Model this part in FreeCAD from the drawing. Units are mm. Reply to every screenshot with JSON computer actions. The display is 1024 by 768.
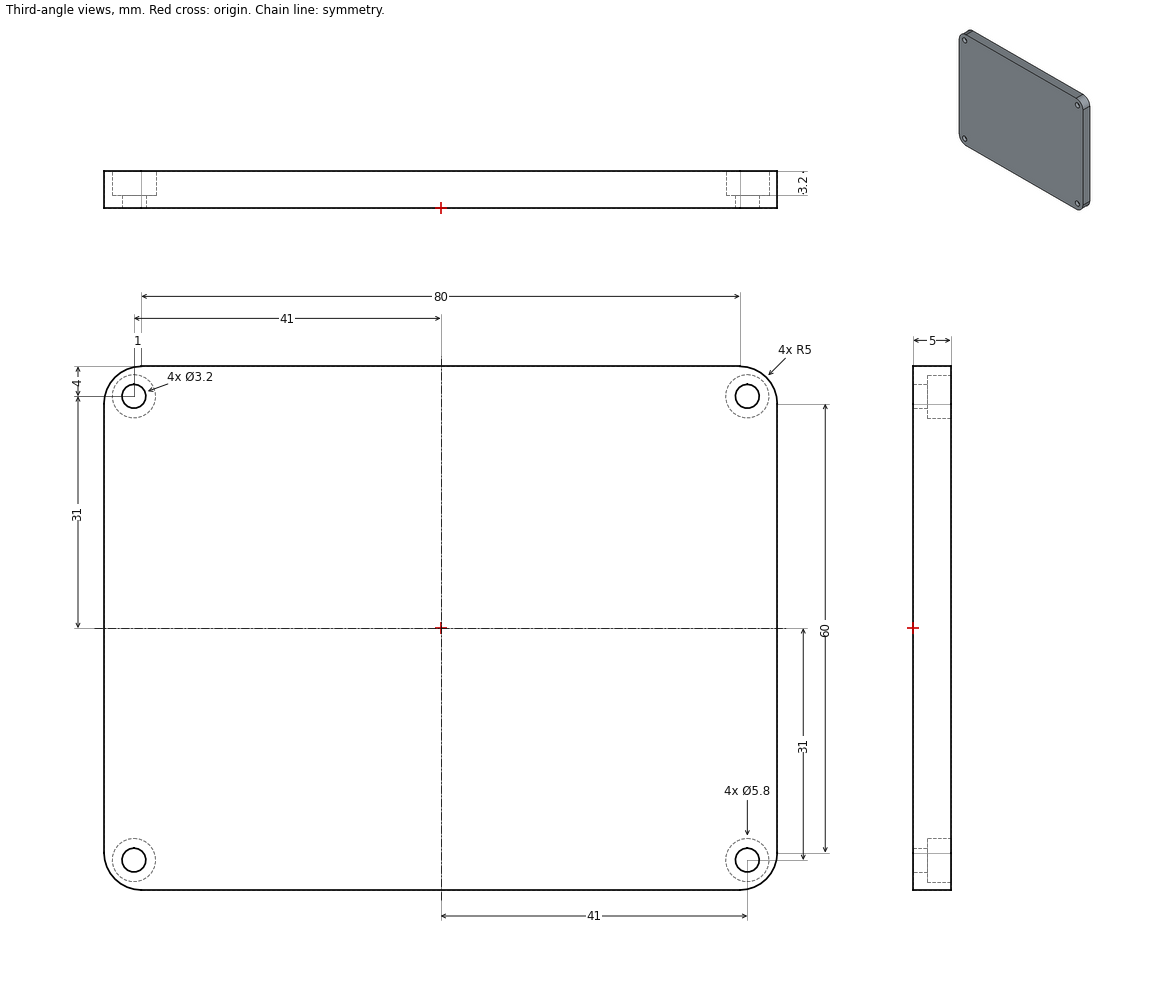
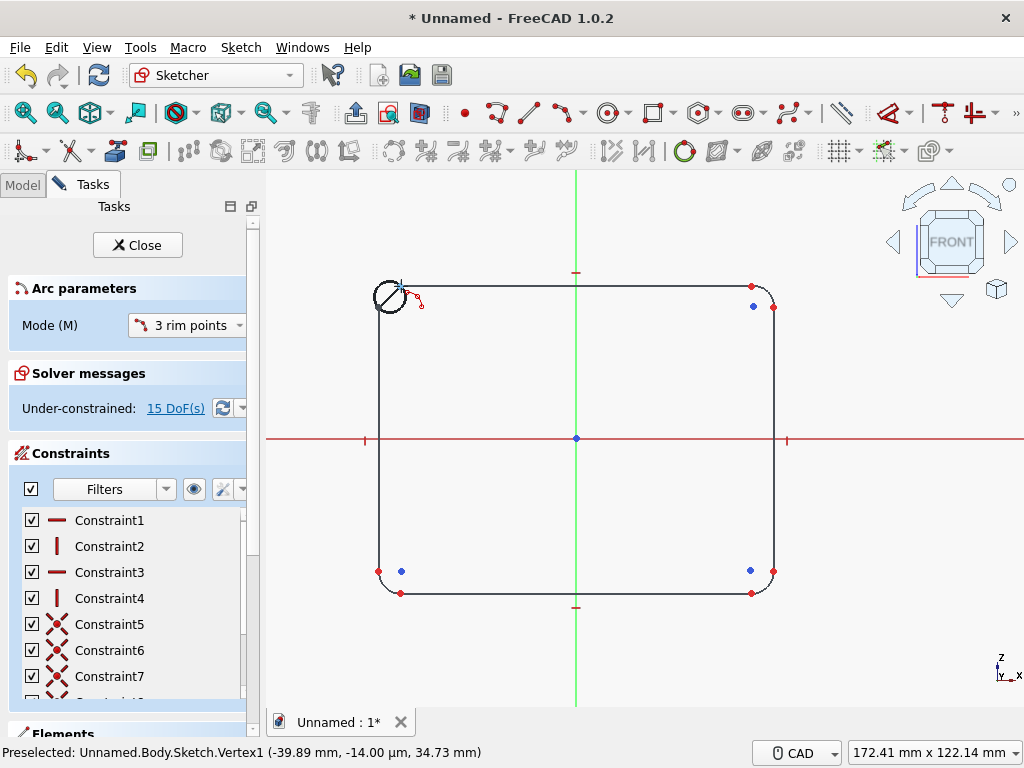
{"action": "scroll", "coordinate": [385, 291], "scroll_direction": "up", "scroll_amount": 5}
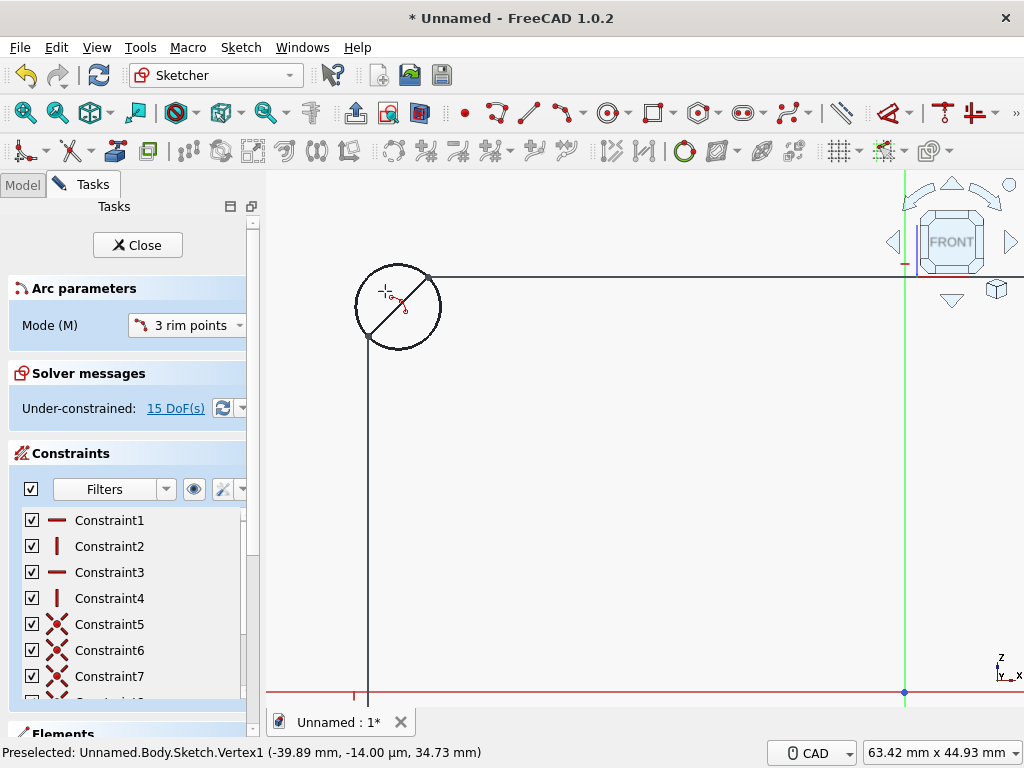
{"action": "left_click", "coordinate": [384, 291]}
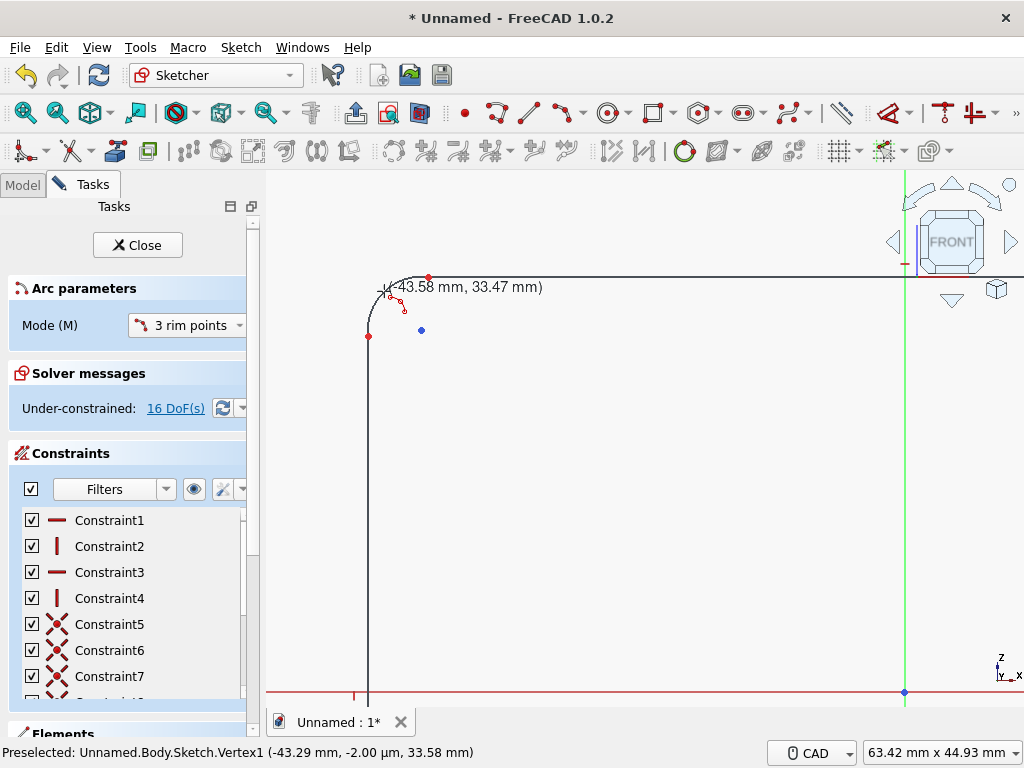
{"action": "key", "text": "g c"}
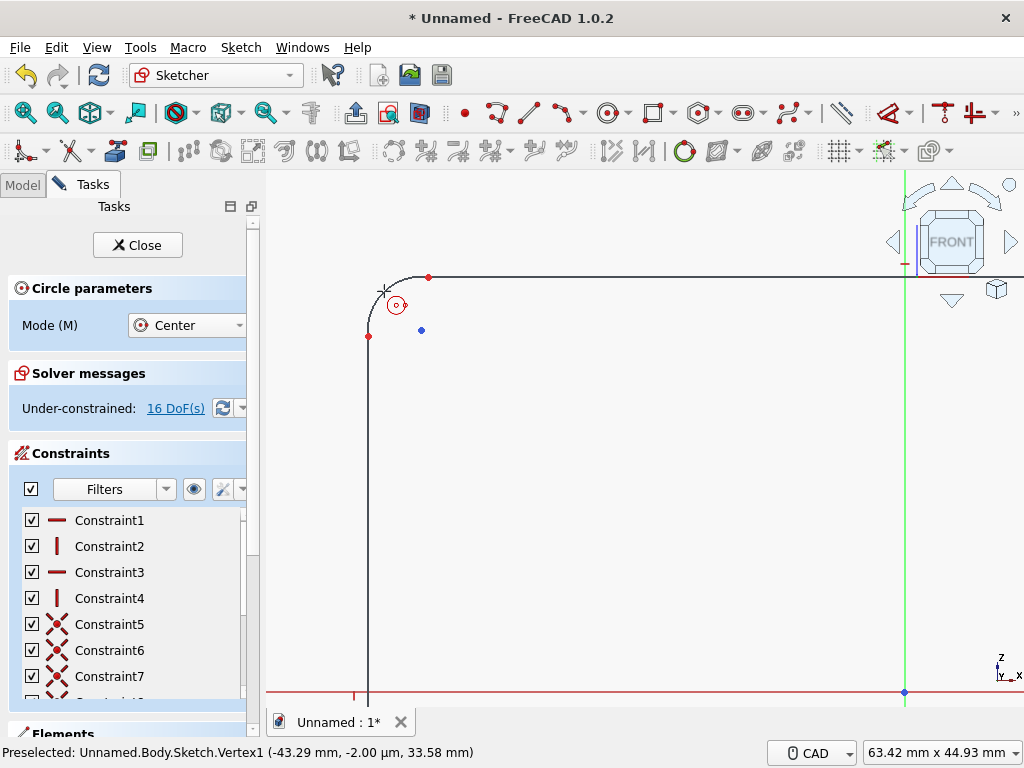
{"action": "left_click", "coordinate": [415, 322]}
{"action": "mouse_move", "coordinate": [428, 308]}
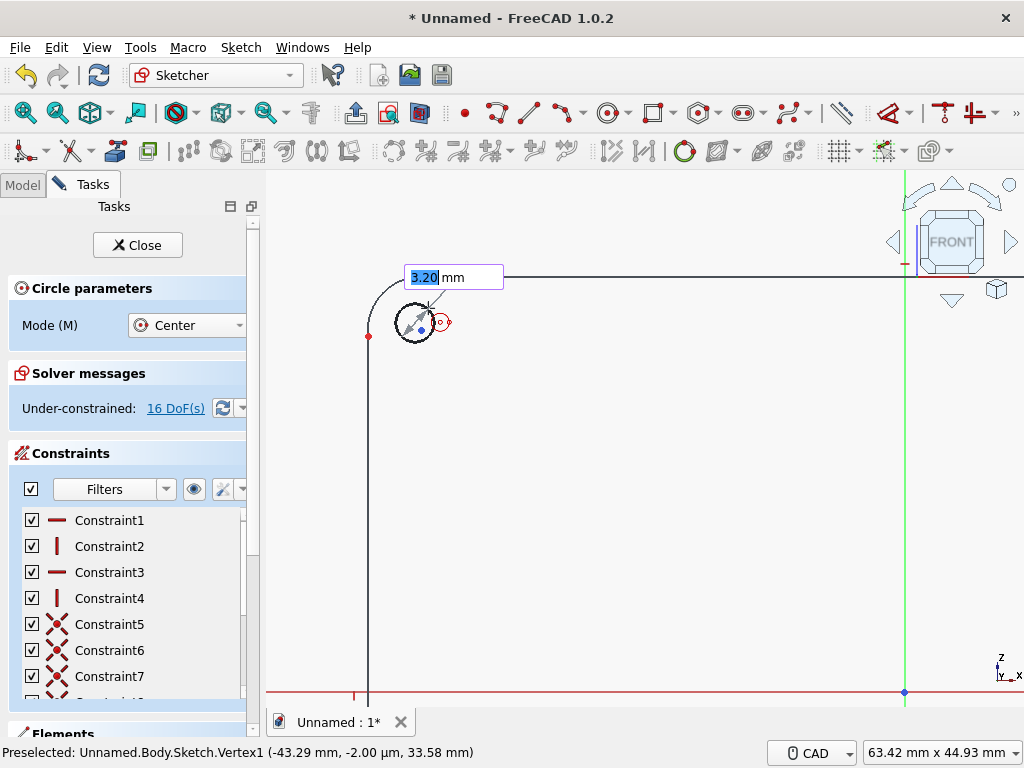
{"action": "type", "text": "3.2"}
{"action": "key", "text": "Return"}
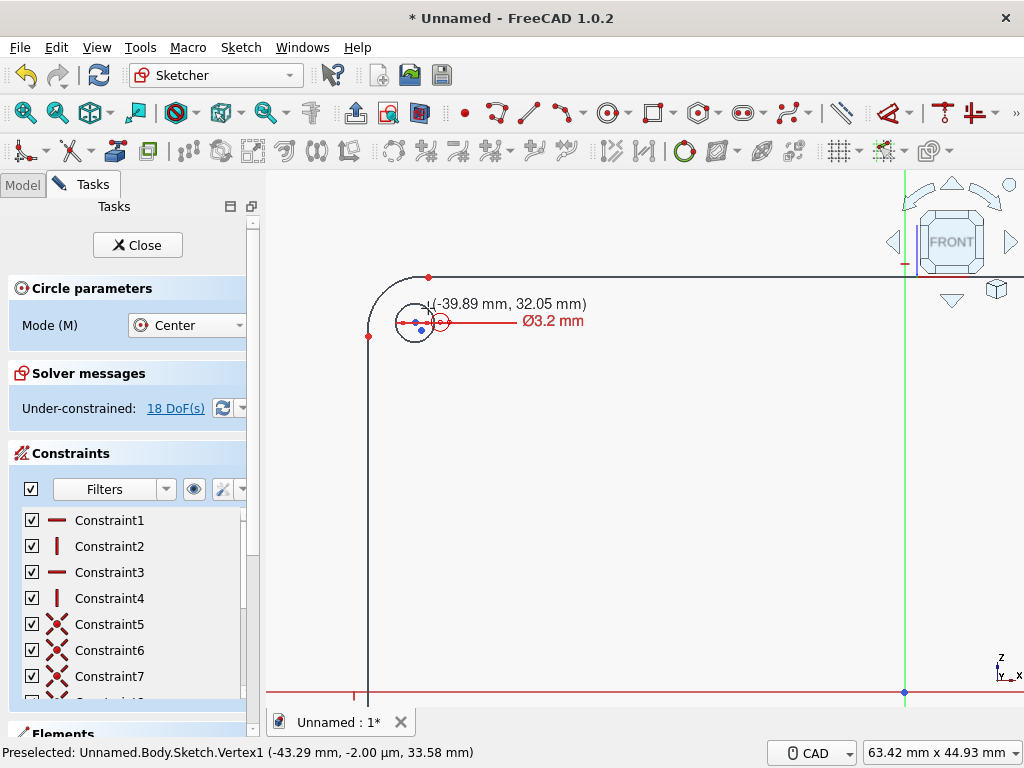
{"action": "scroll", "coordinate": [385, 291], "scroll_direction": "down", "scroll_amount": 5}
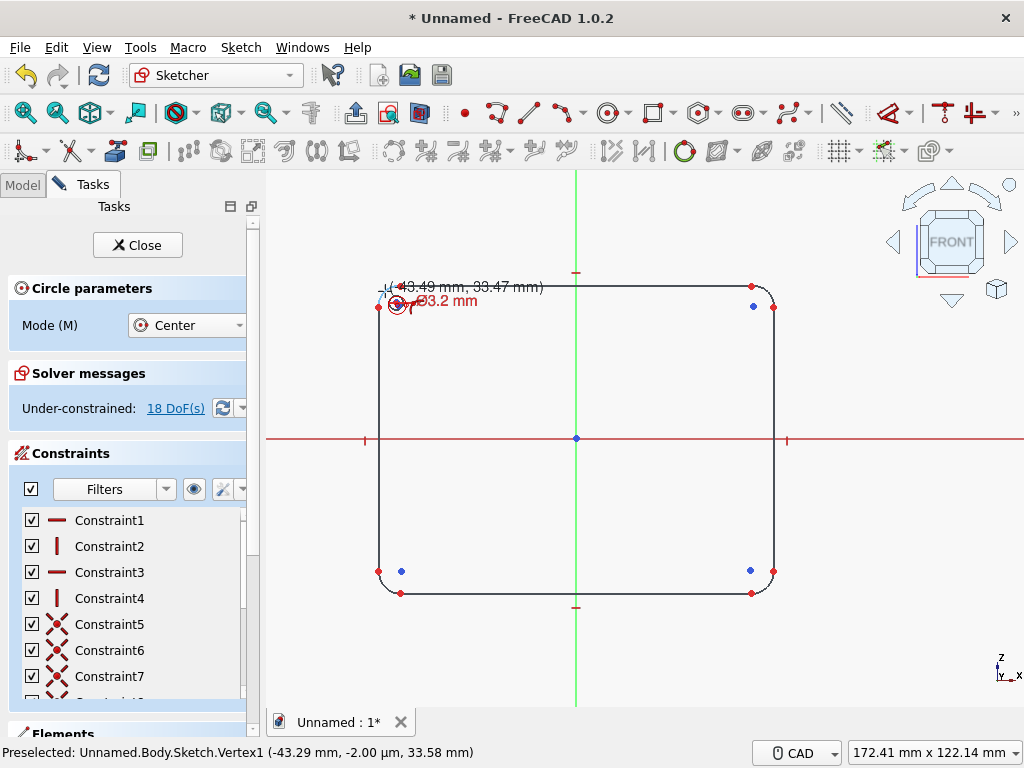
{"action": "scroll", "coordinate": [757, 302], "scroll_direction": "up", "scroll_amount": 6}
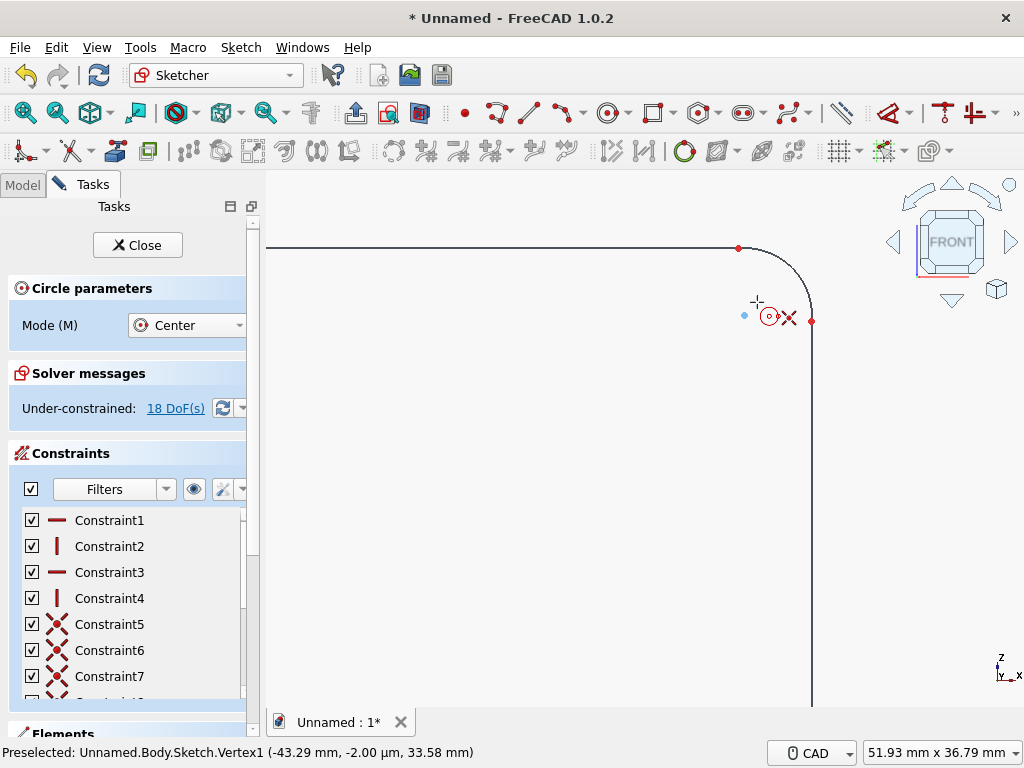
{"action": "left_click", "coordinate": [754, 303]}
{"action": "mouse_move", "coordinate": [771, 286]}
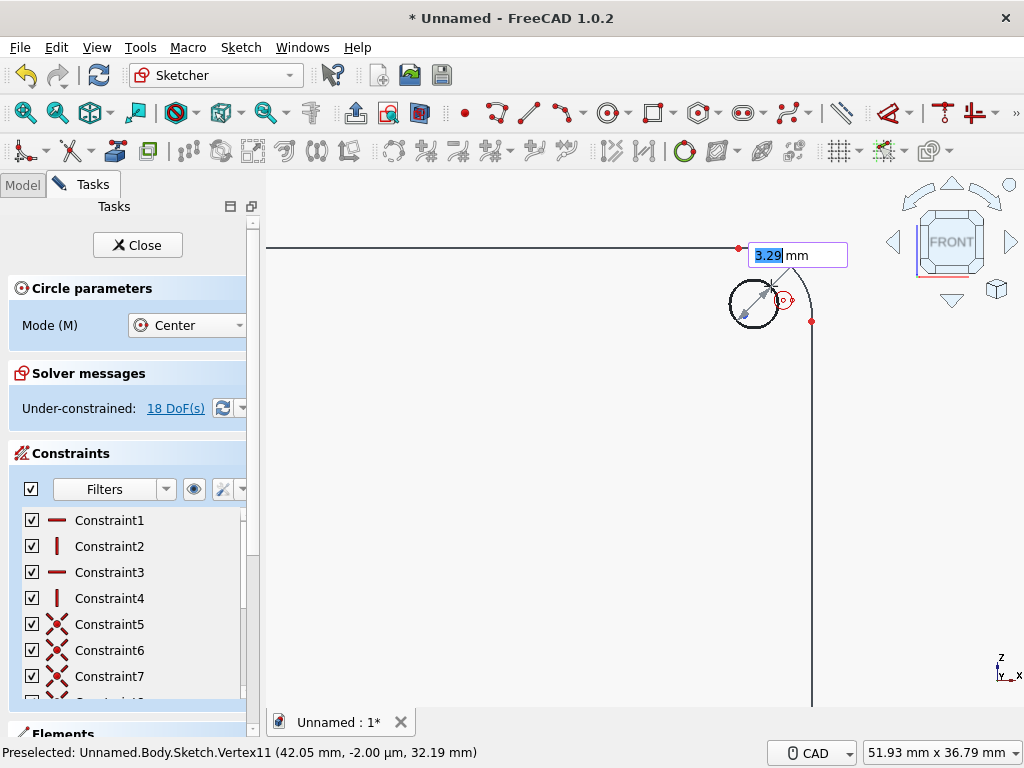
{"action": "type", "text": "3.2"}
{"action": "key", "text": "Return"}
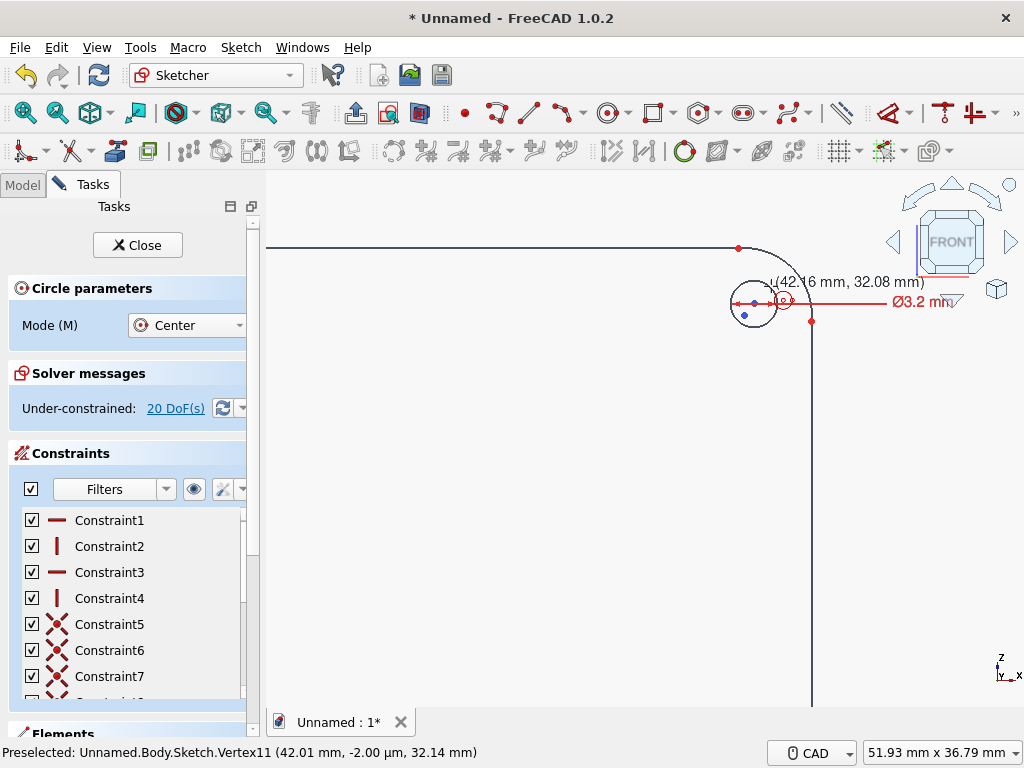
{"action": "scroll", "coordinate": [758, 302], "scroll_direction": "down", "scroll_amount": 6}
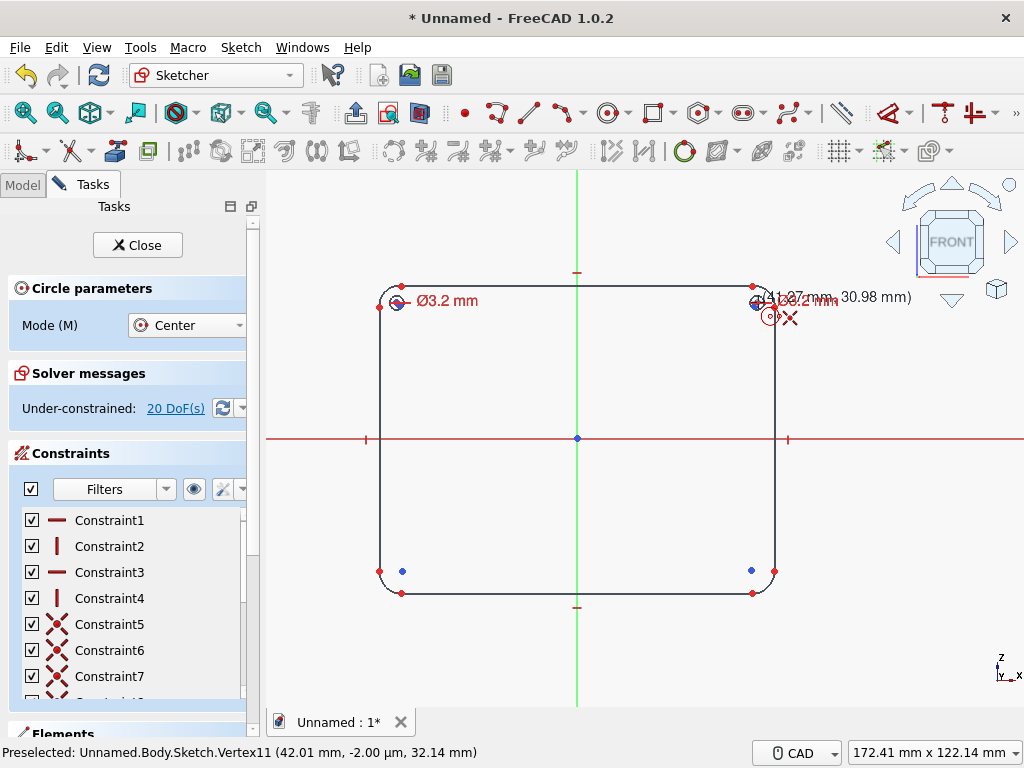
{"action": "scroll", "coordinate": [397, 575], "scroll_direction": "up", "scroll_amount": 6}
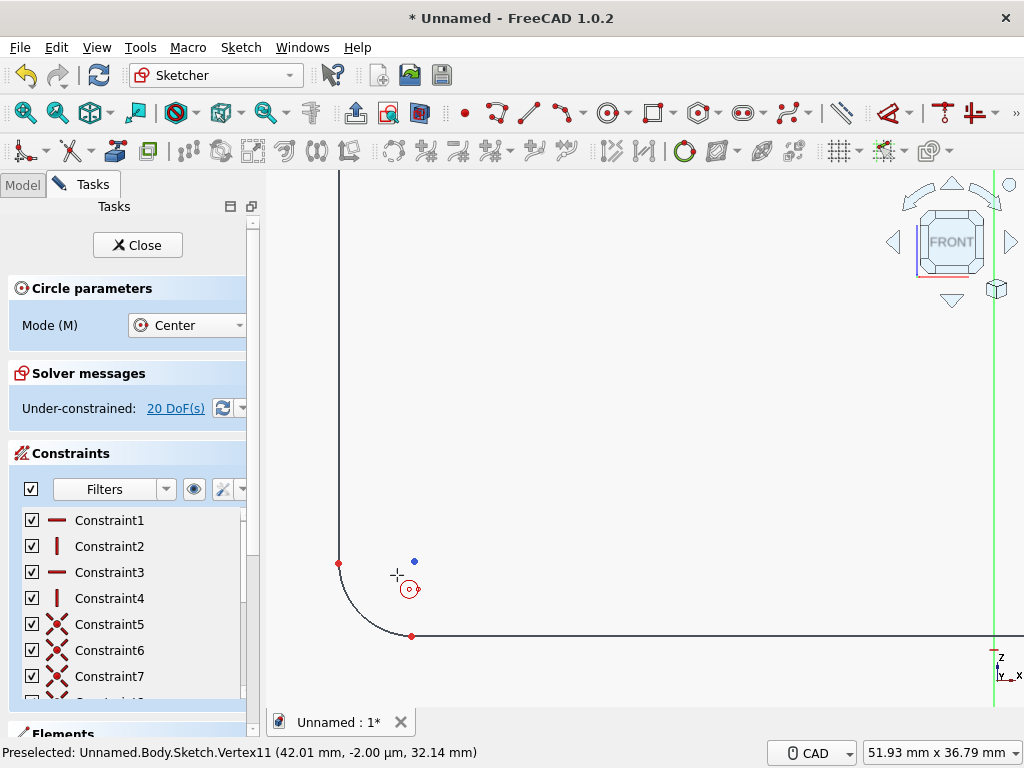
{"action": "left_click", "coordinate": [396, 573]}
{"action": "mouse_move", "coordinate": [379, 557]}